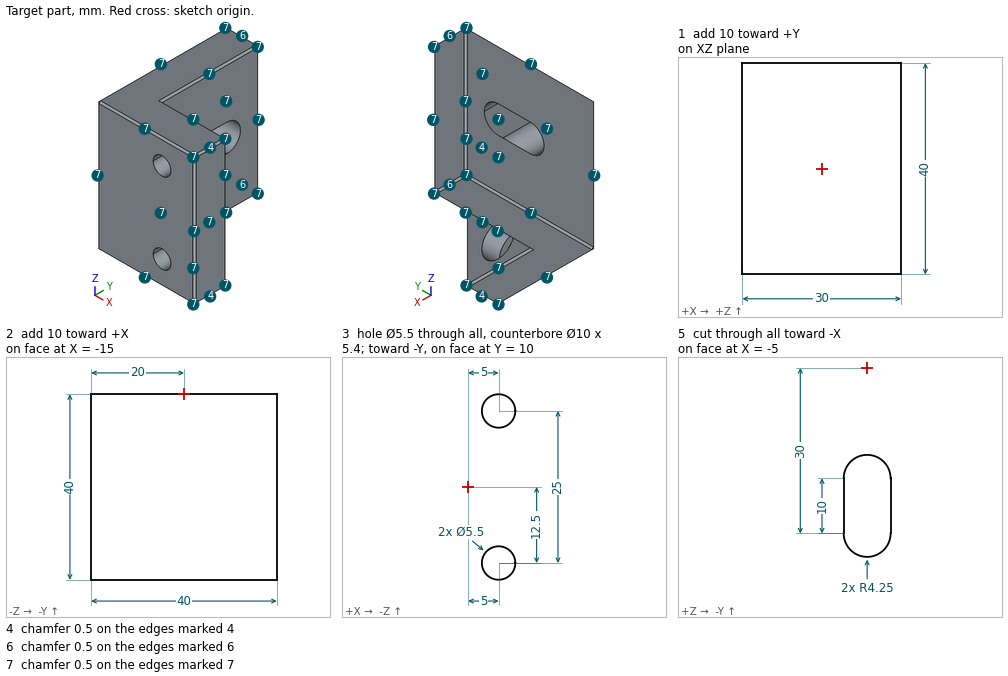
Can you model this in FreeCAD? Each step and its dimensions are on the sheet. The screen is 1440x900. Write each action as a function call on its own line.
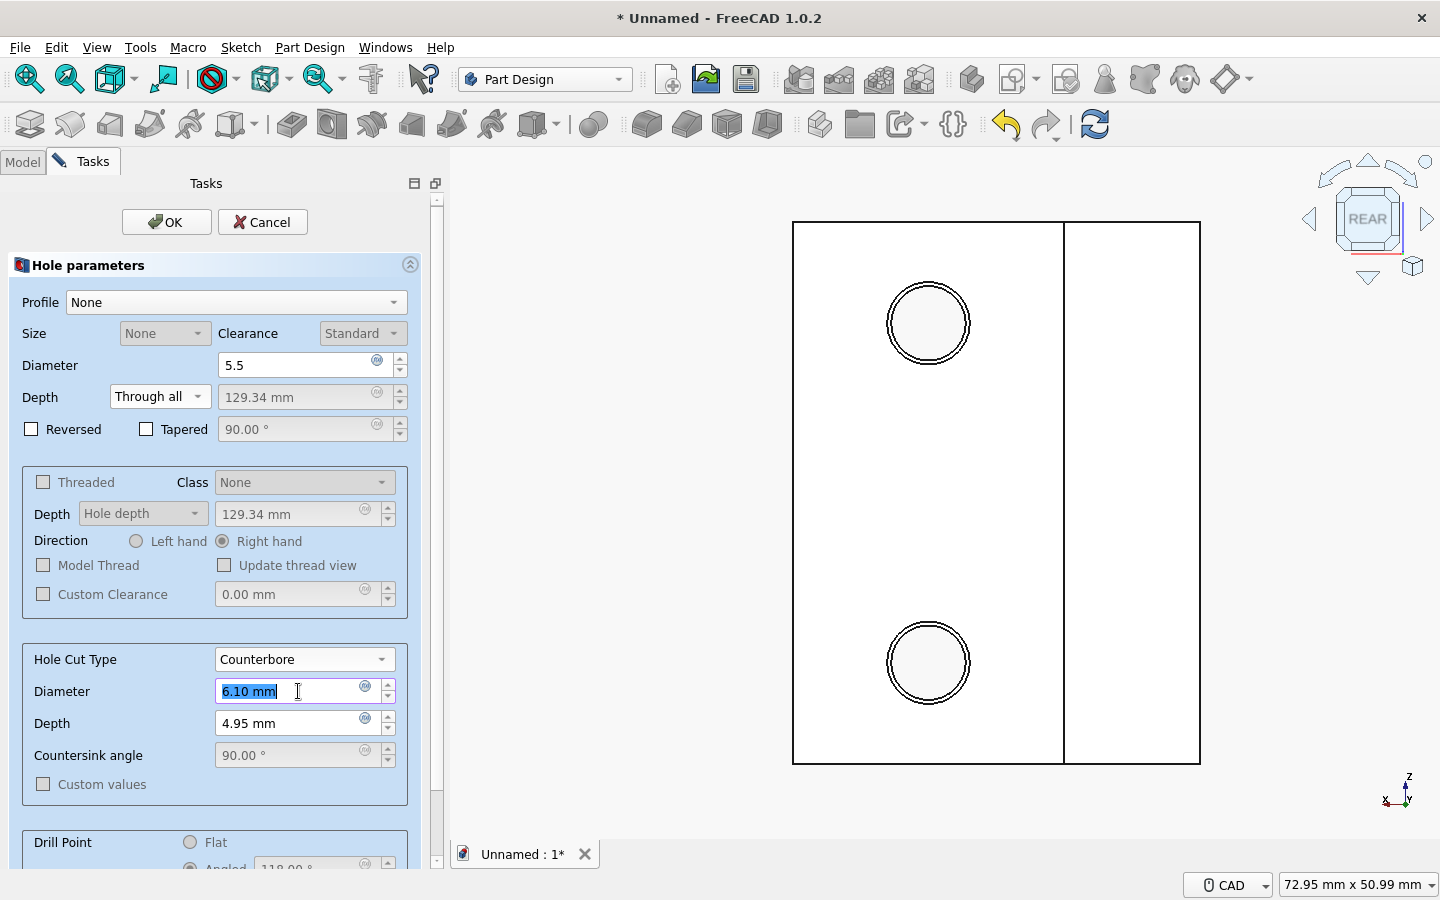
text(10)
key(Tab)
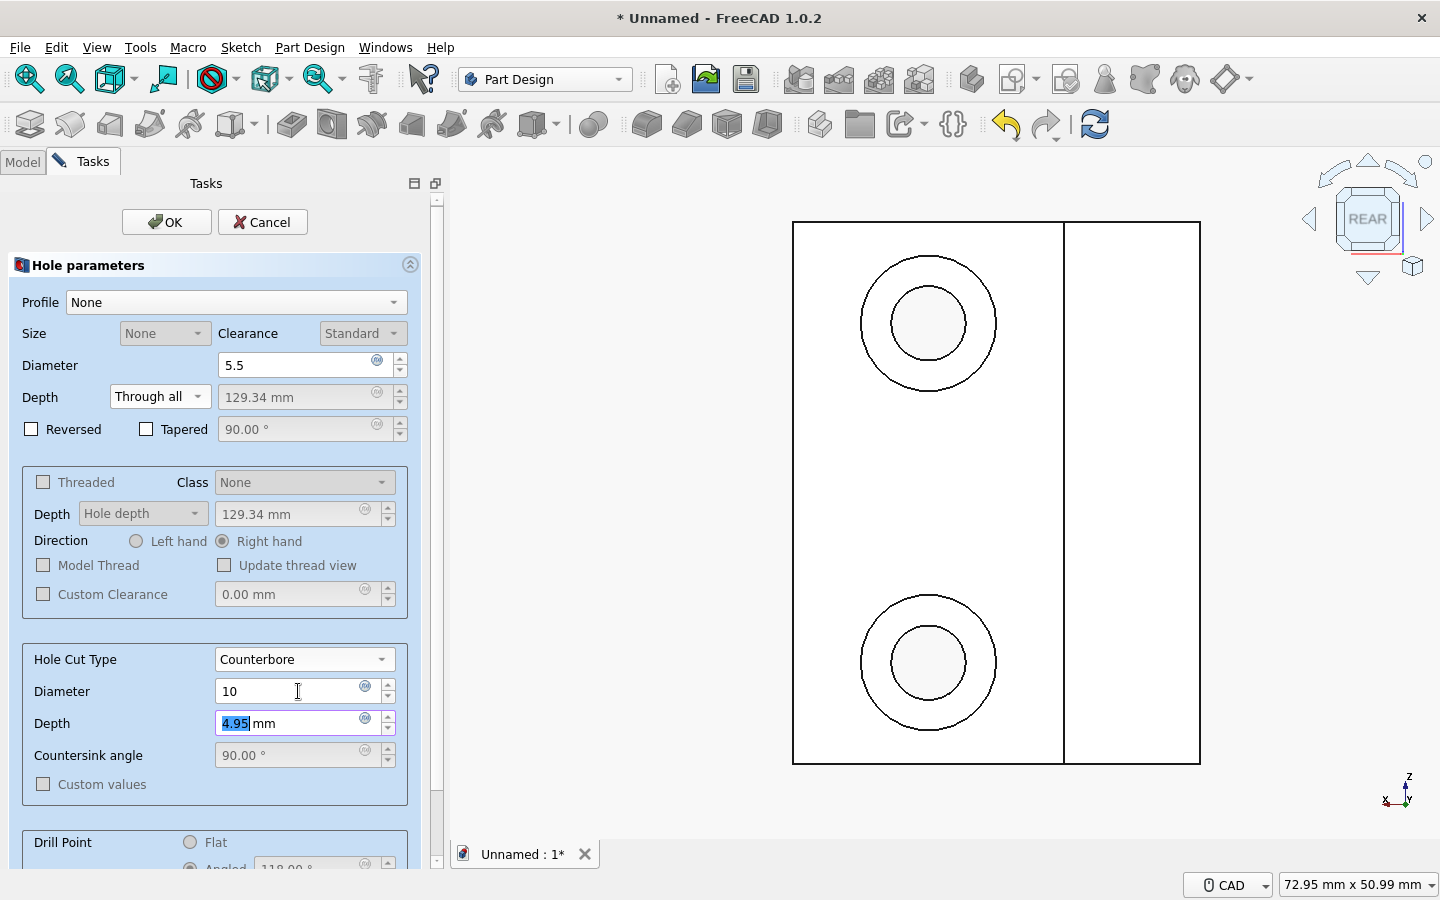
text(5.4)
key(Tab)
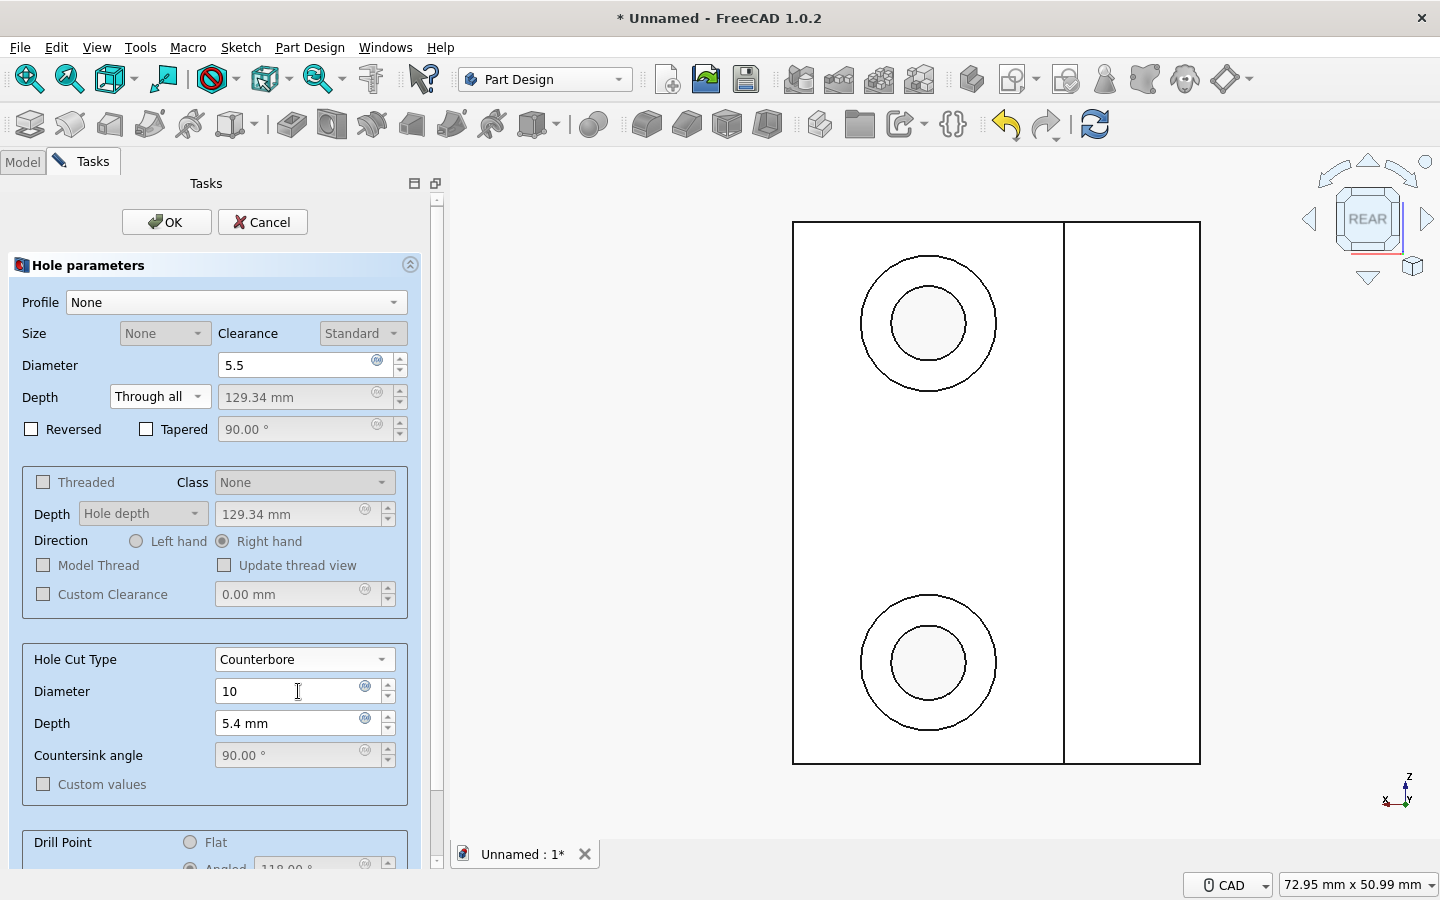
click(167, 222)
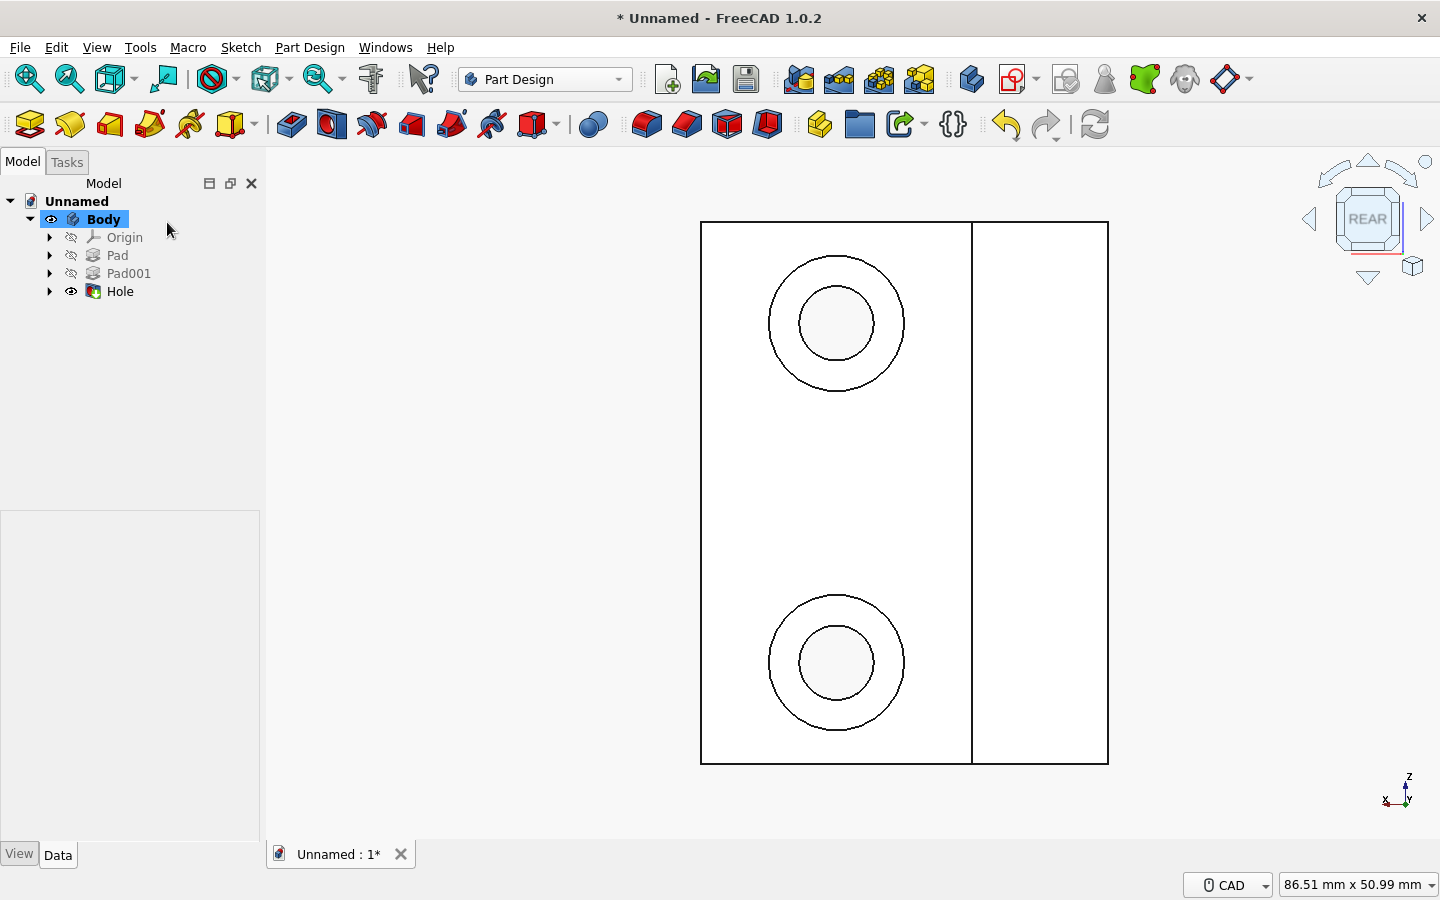
key(0)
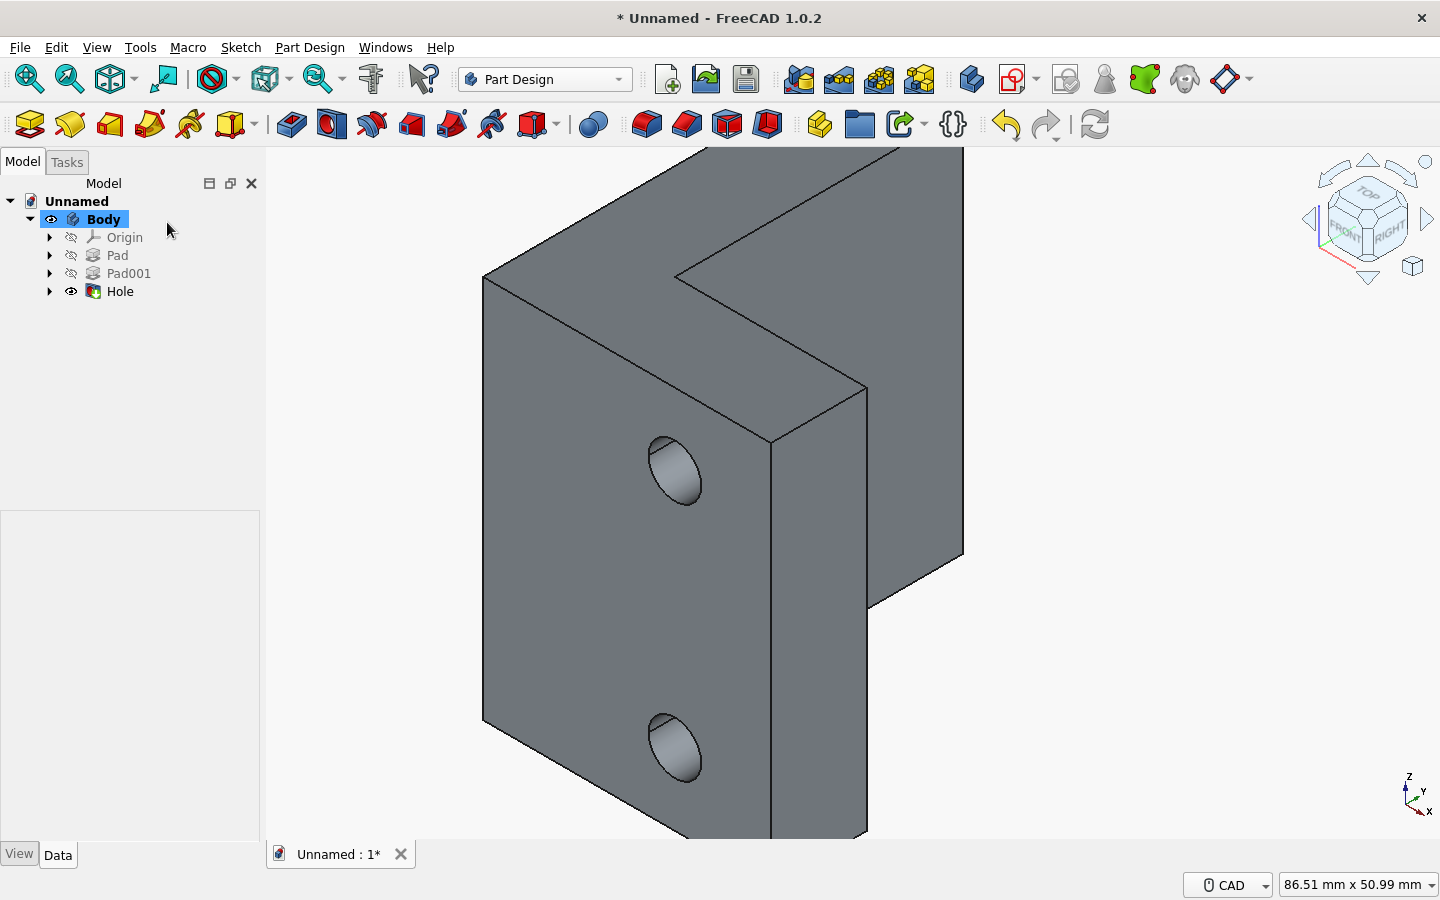
click(30, 80)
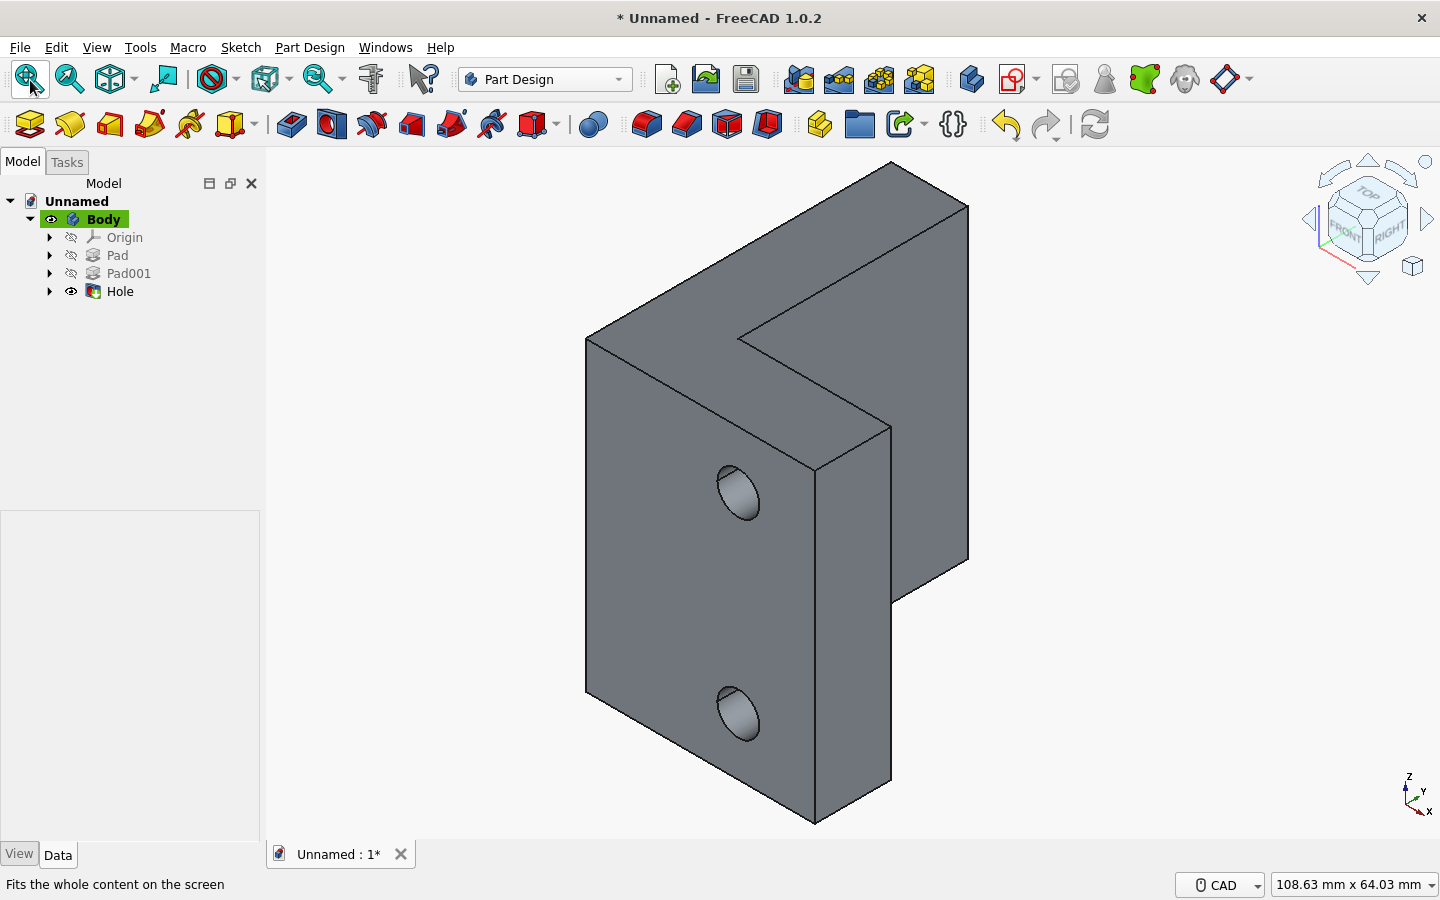
click(853, 448)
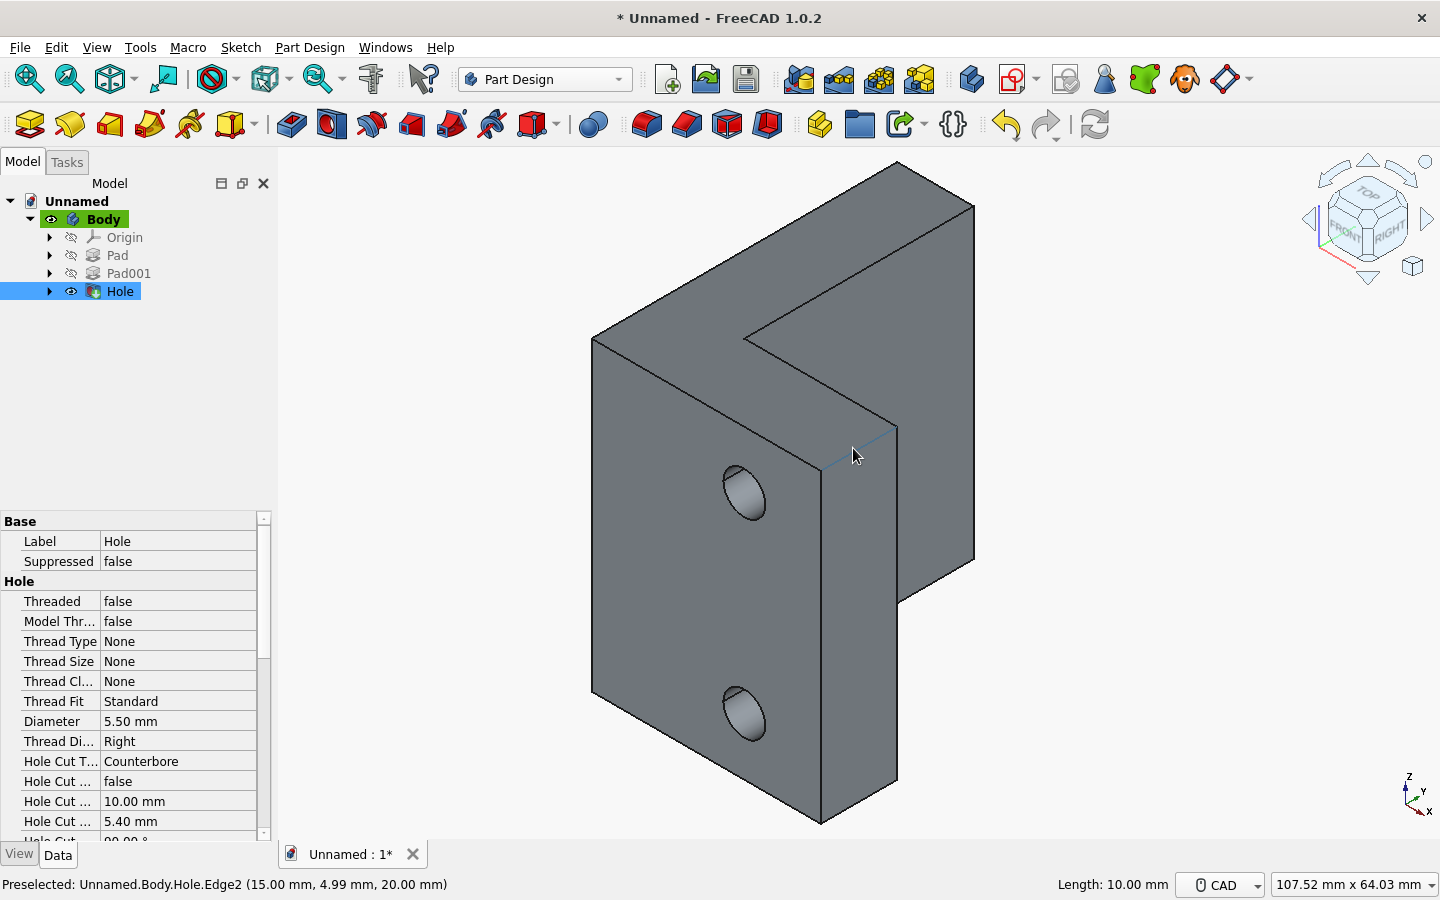
key(2)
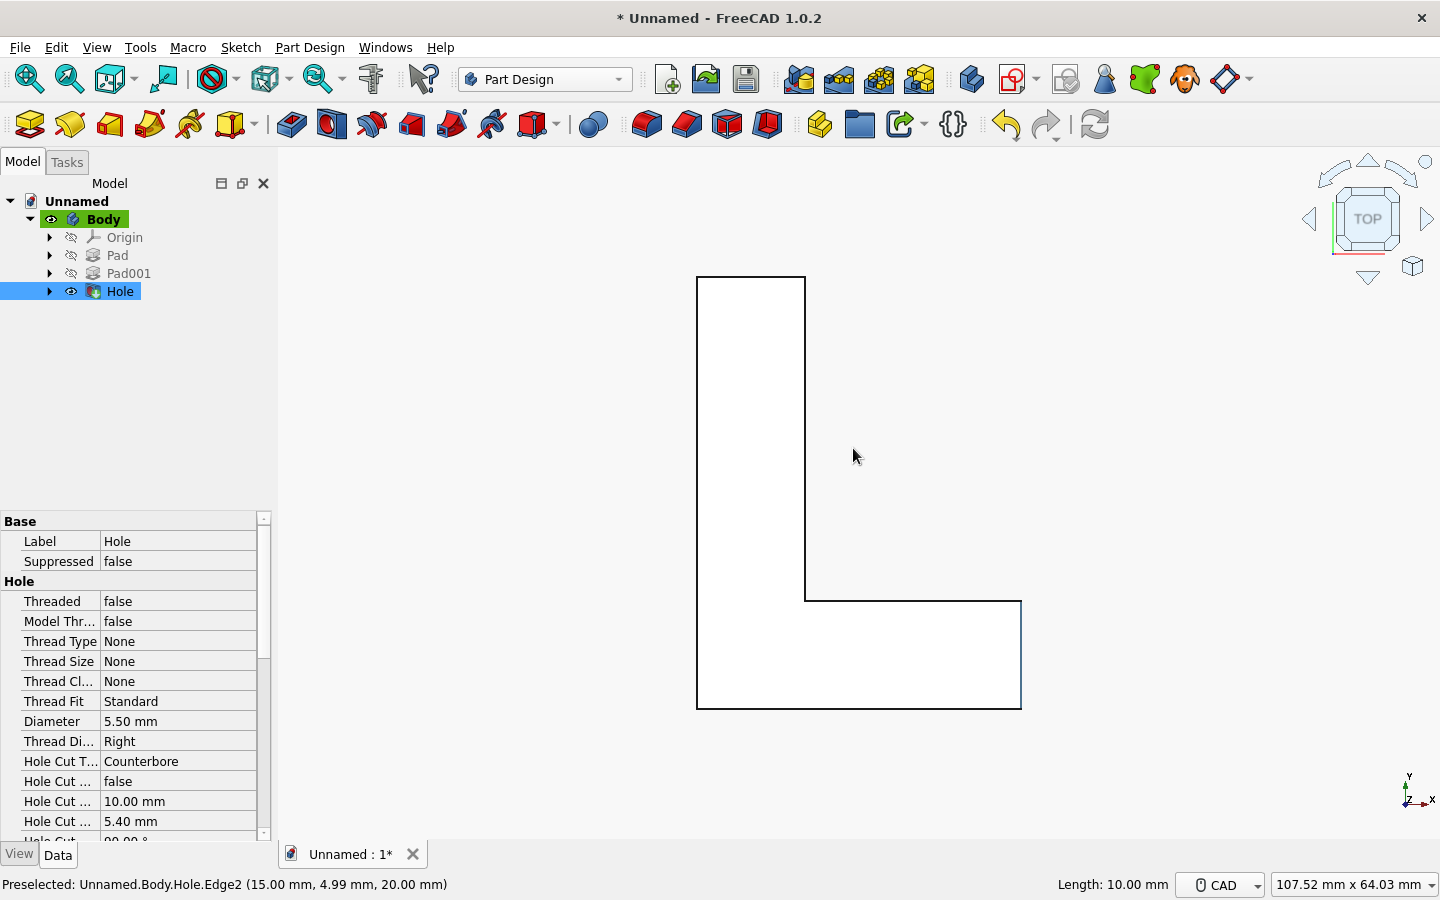
key(1)